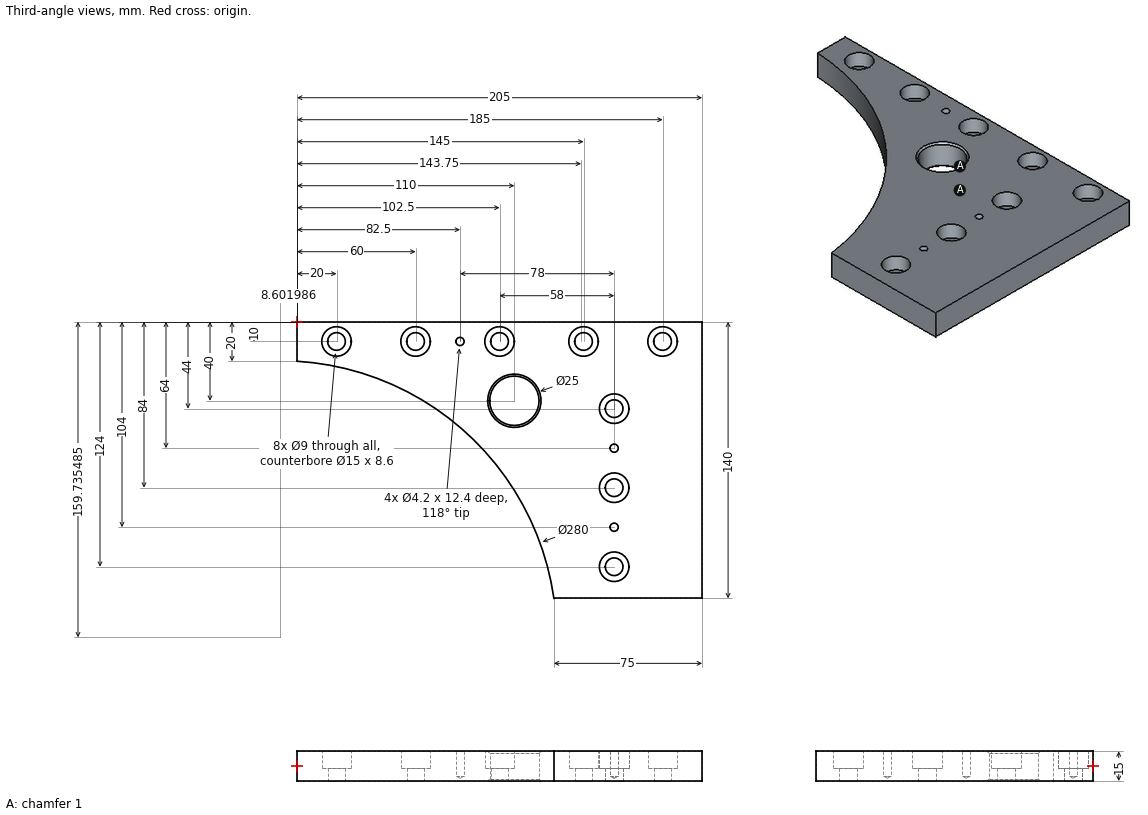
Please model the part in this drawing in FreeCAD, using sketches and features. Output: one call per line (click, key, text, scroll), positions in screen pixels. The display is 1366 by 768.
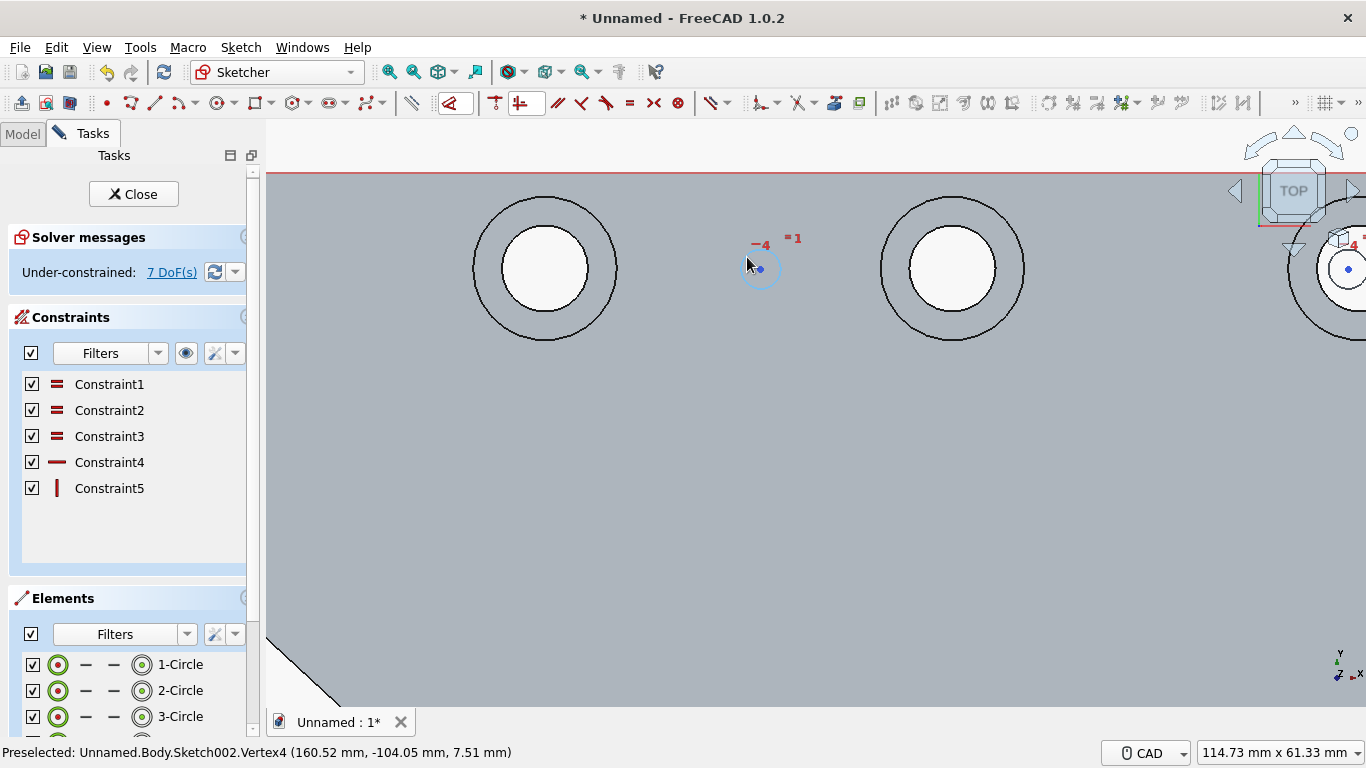
click(747, 255)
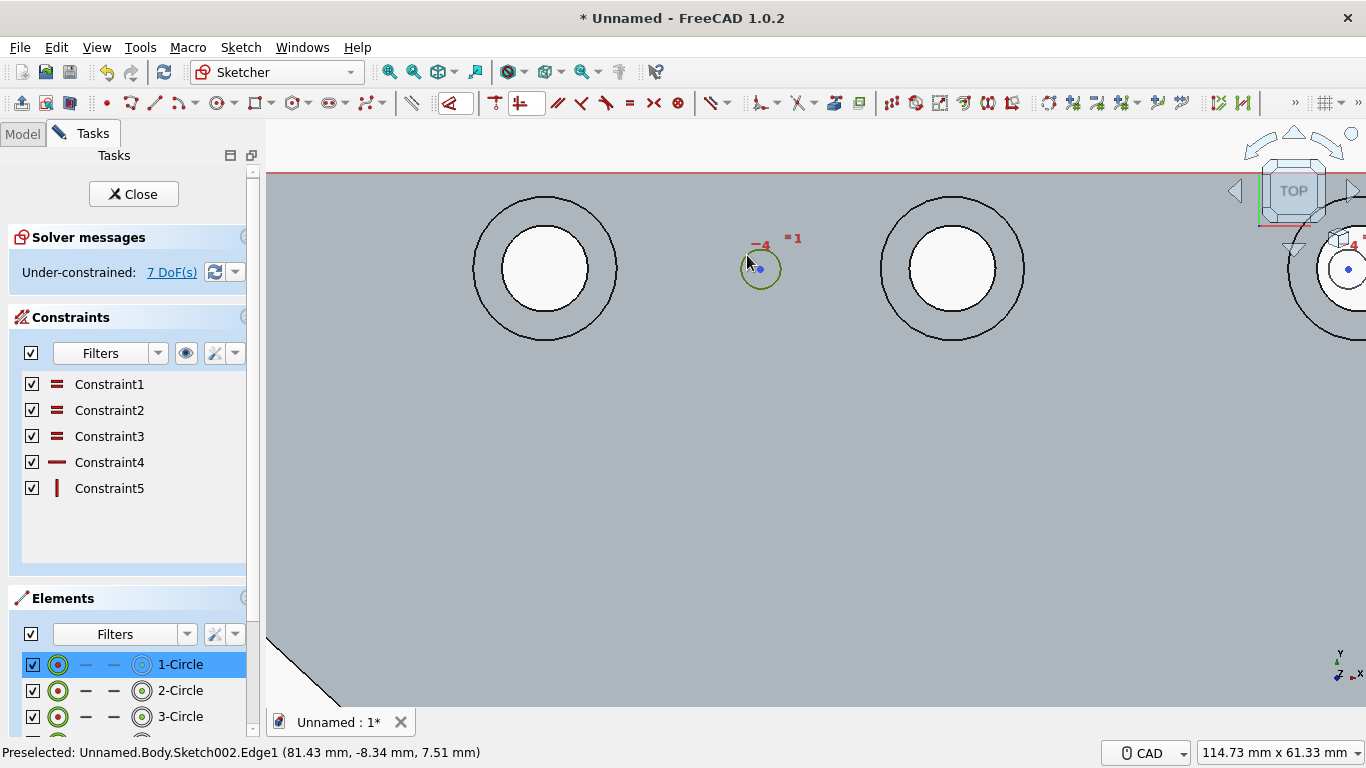
click(468, 104)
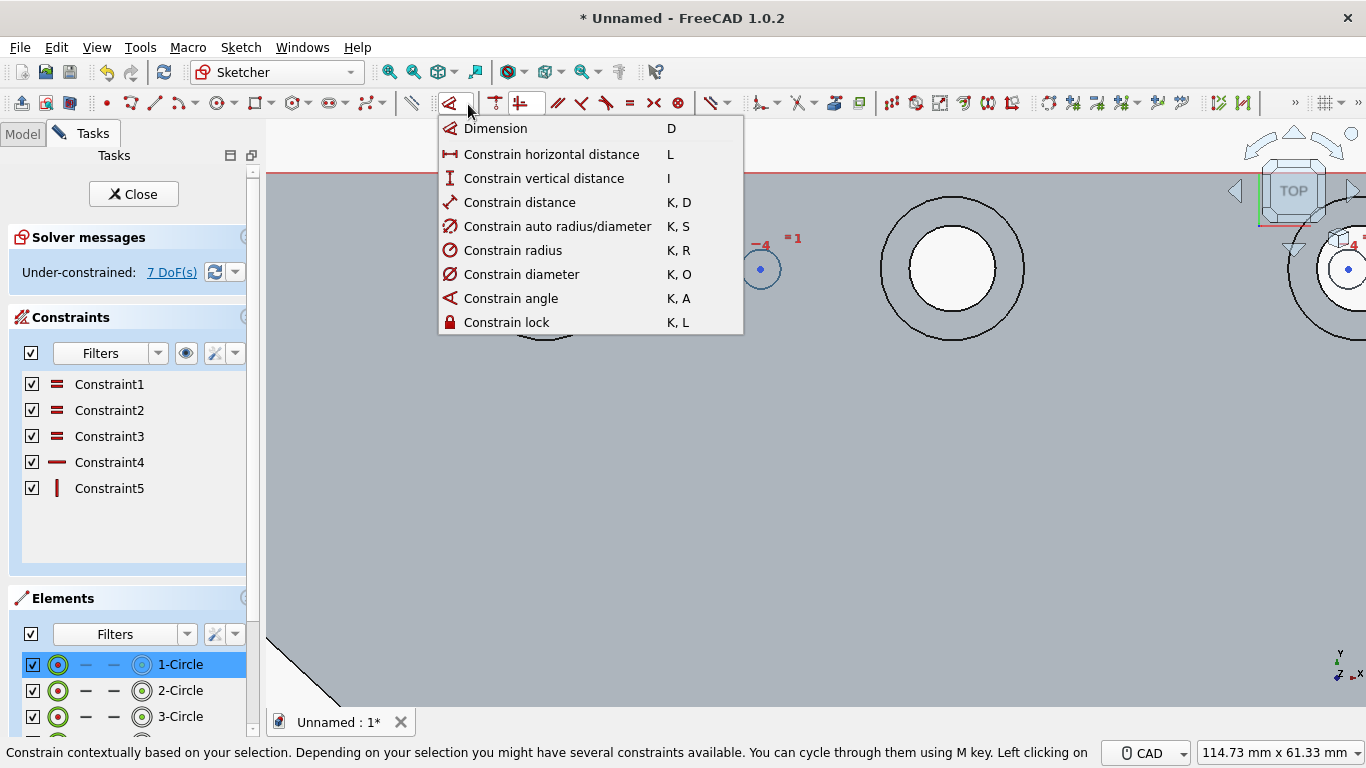
click(591, 274)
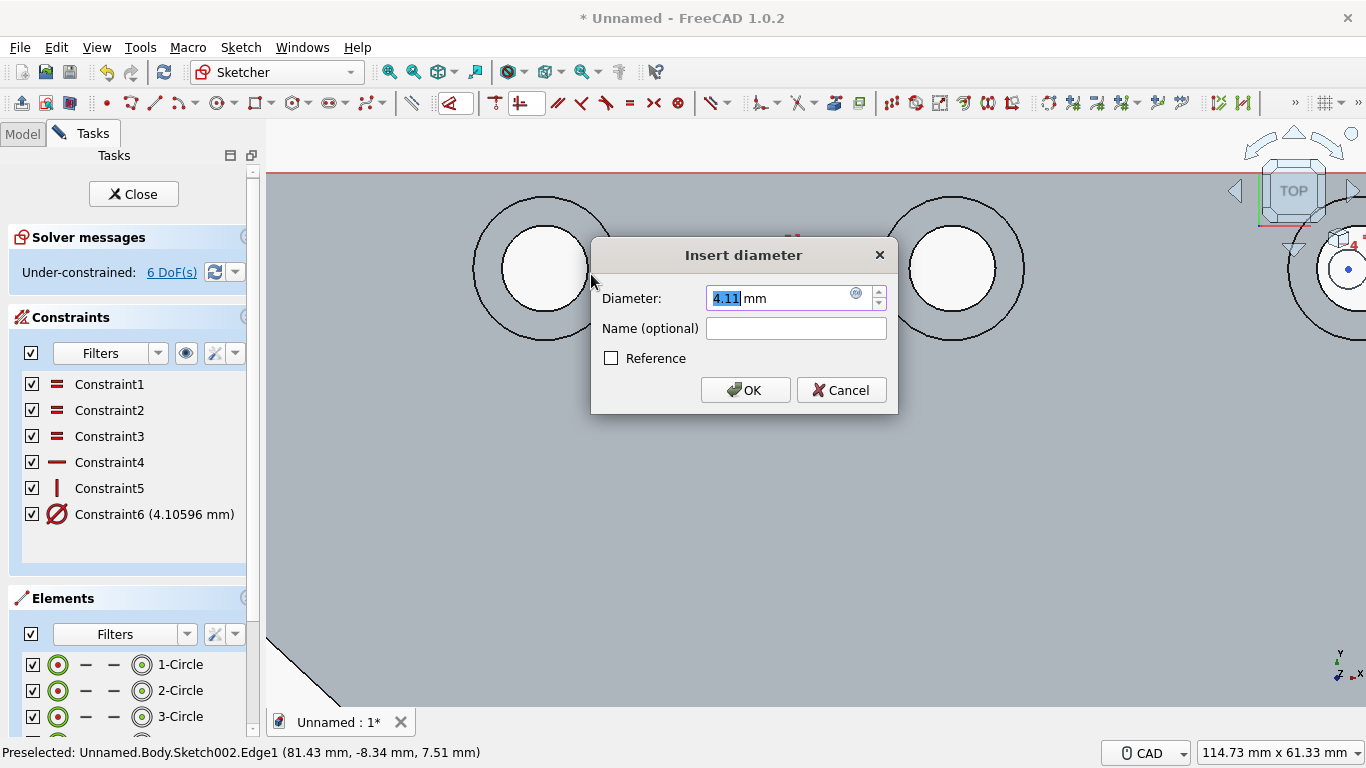
text(4.2)
key(Return)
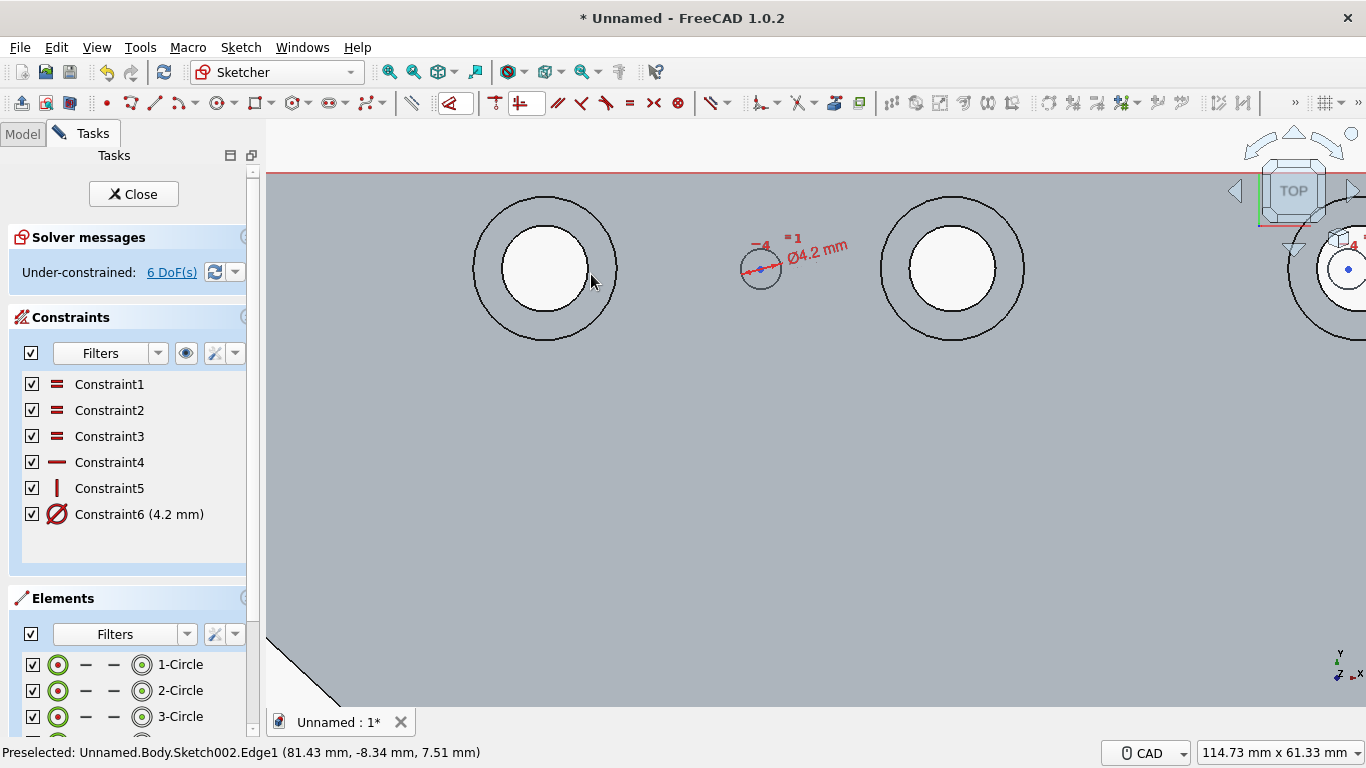
click(761, 269)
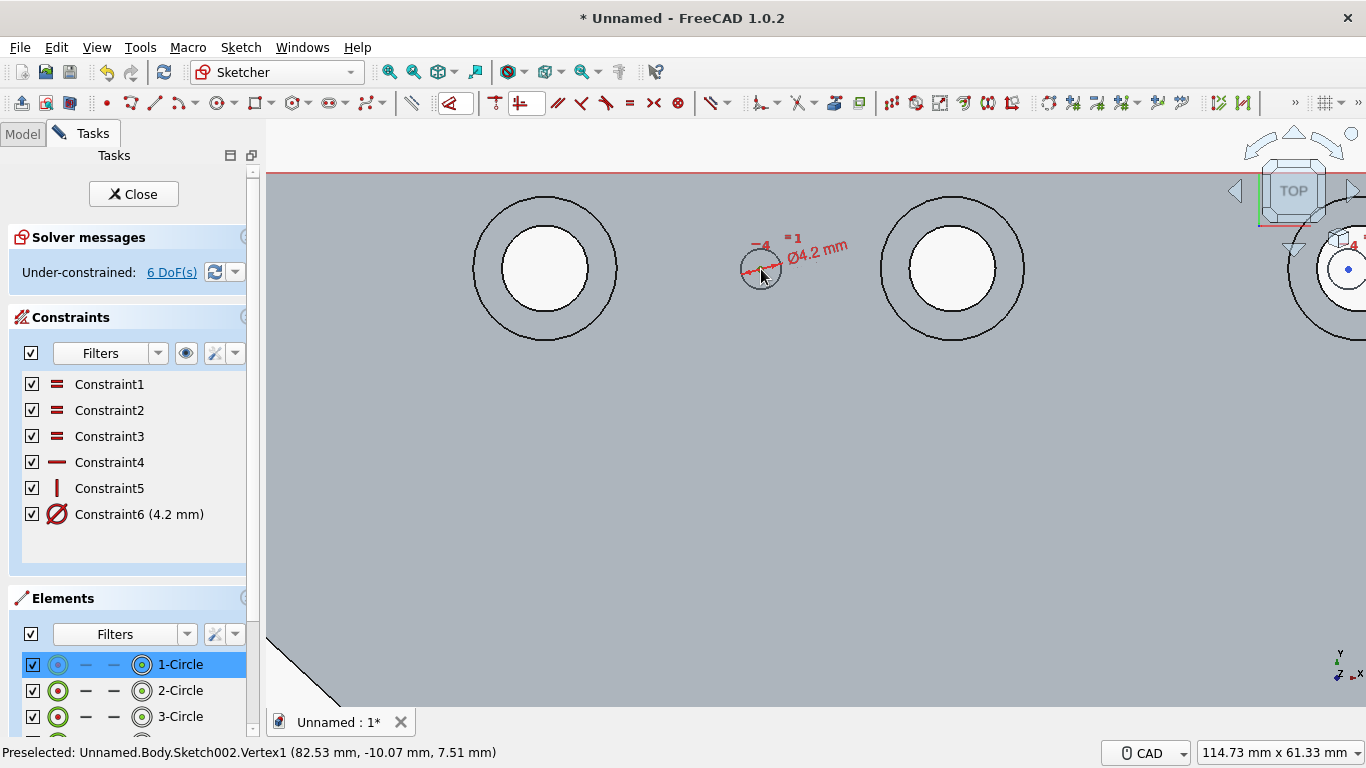
click(468, 104)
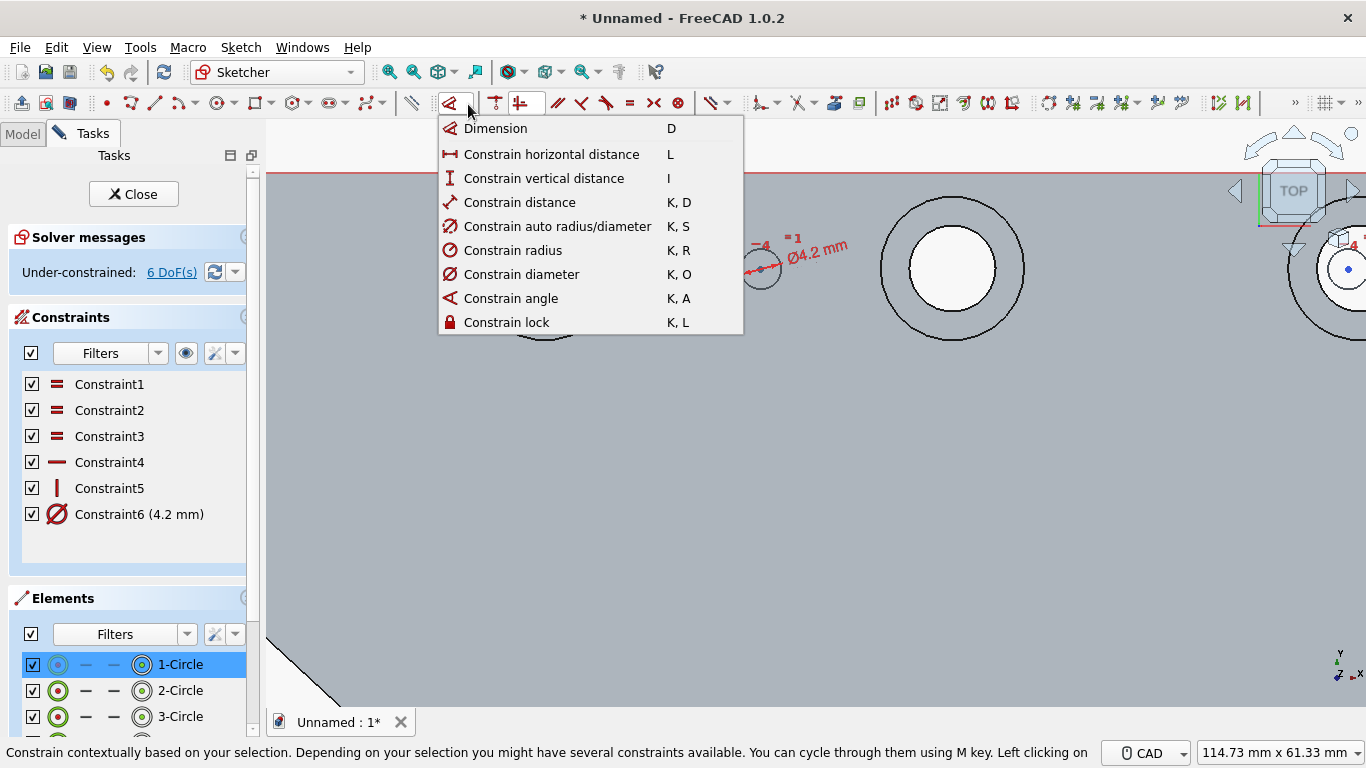
click(591, 178)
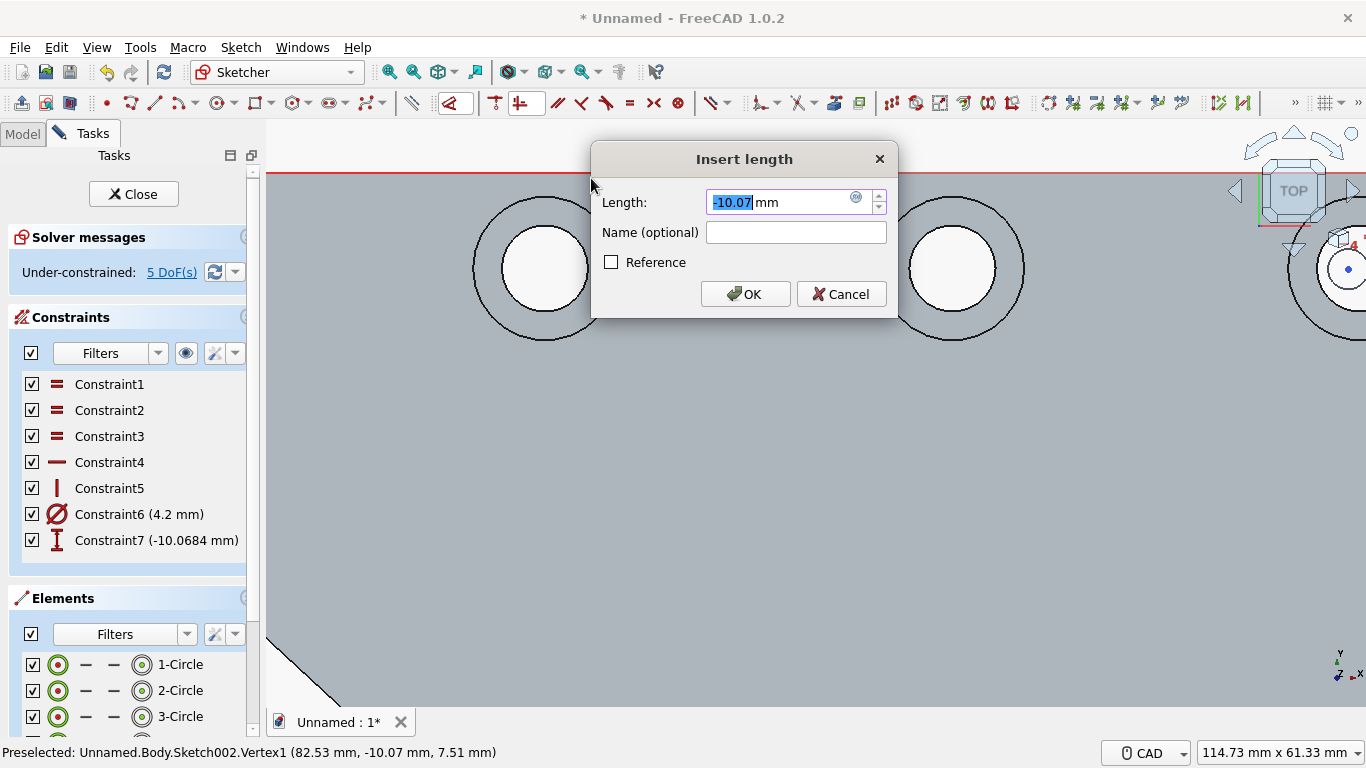
text(-10)
key(Return)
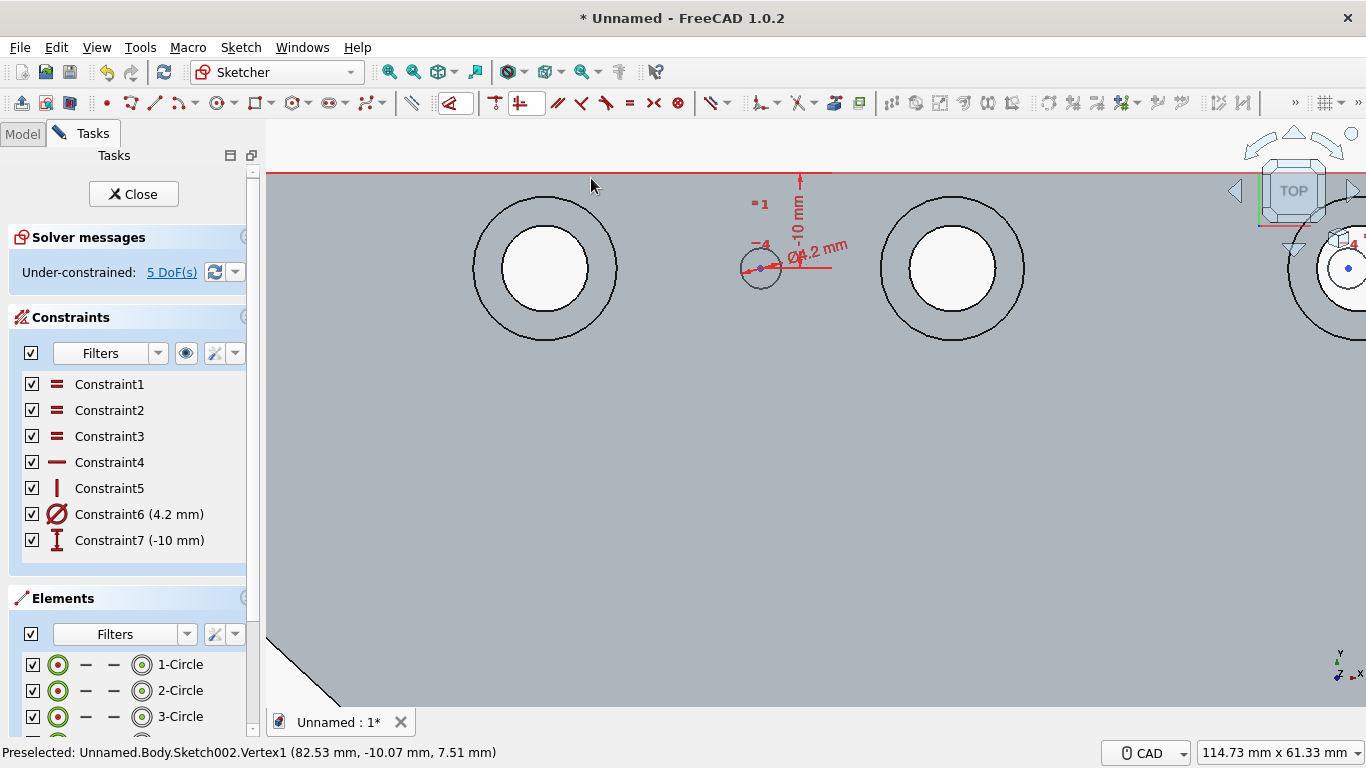
scroll(747, 257, down, 5)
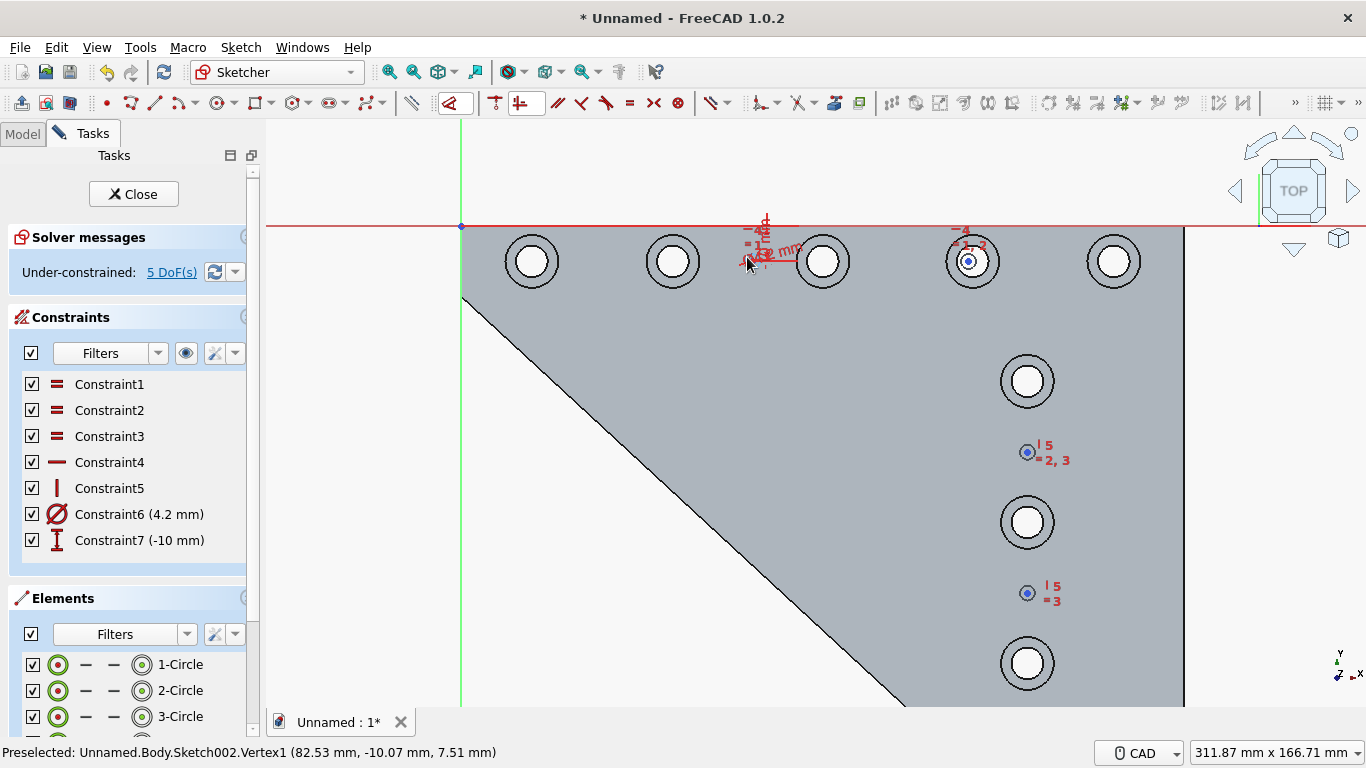
click(1027, 452)